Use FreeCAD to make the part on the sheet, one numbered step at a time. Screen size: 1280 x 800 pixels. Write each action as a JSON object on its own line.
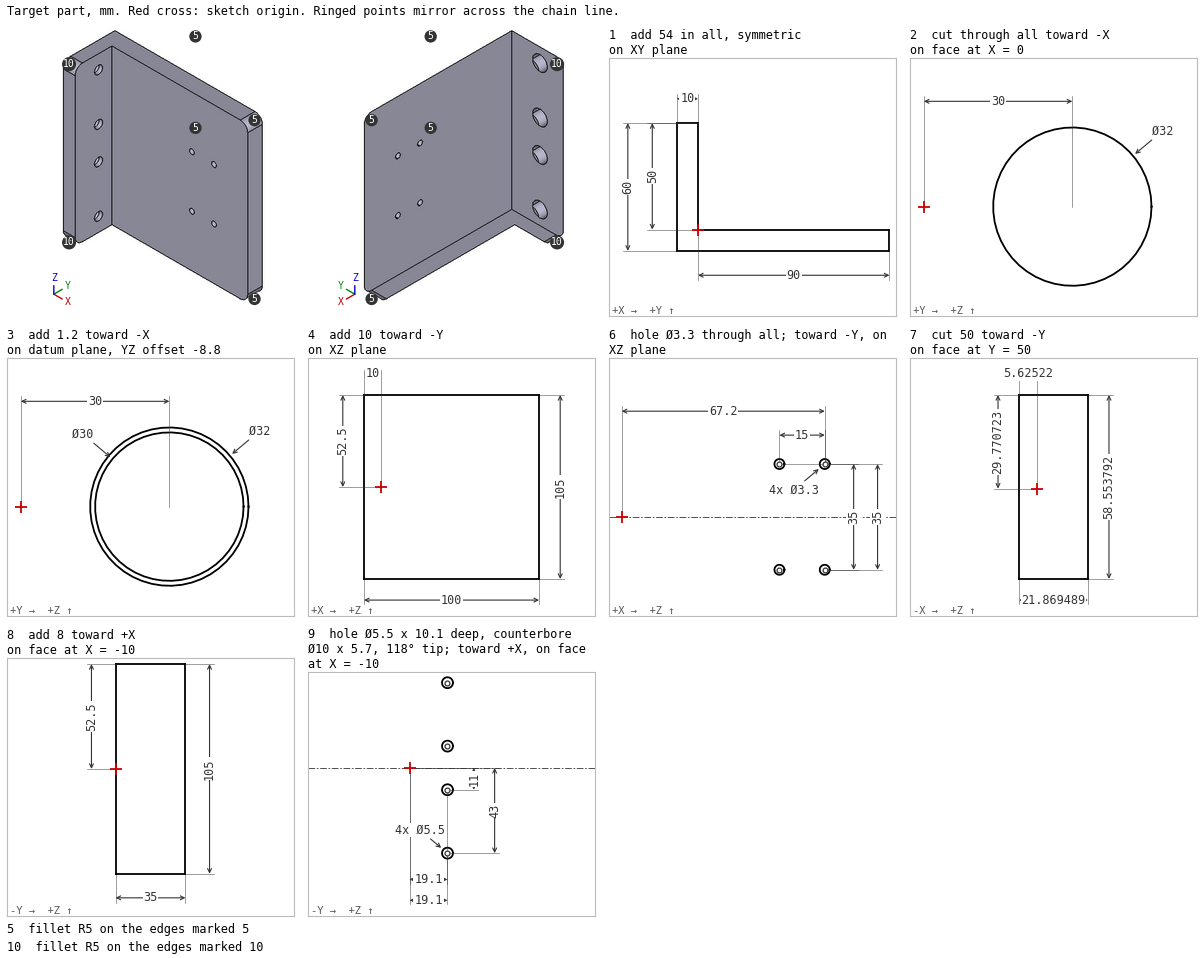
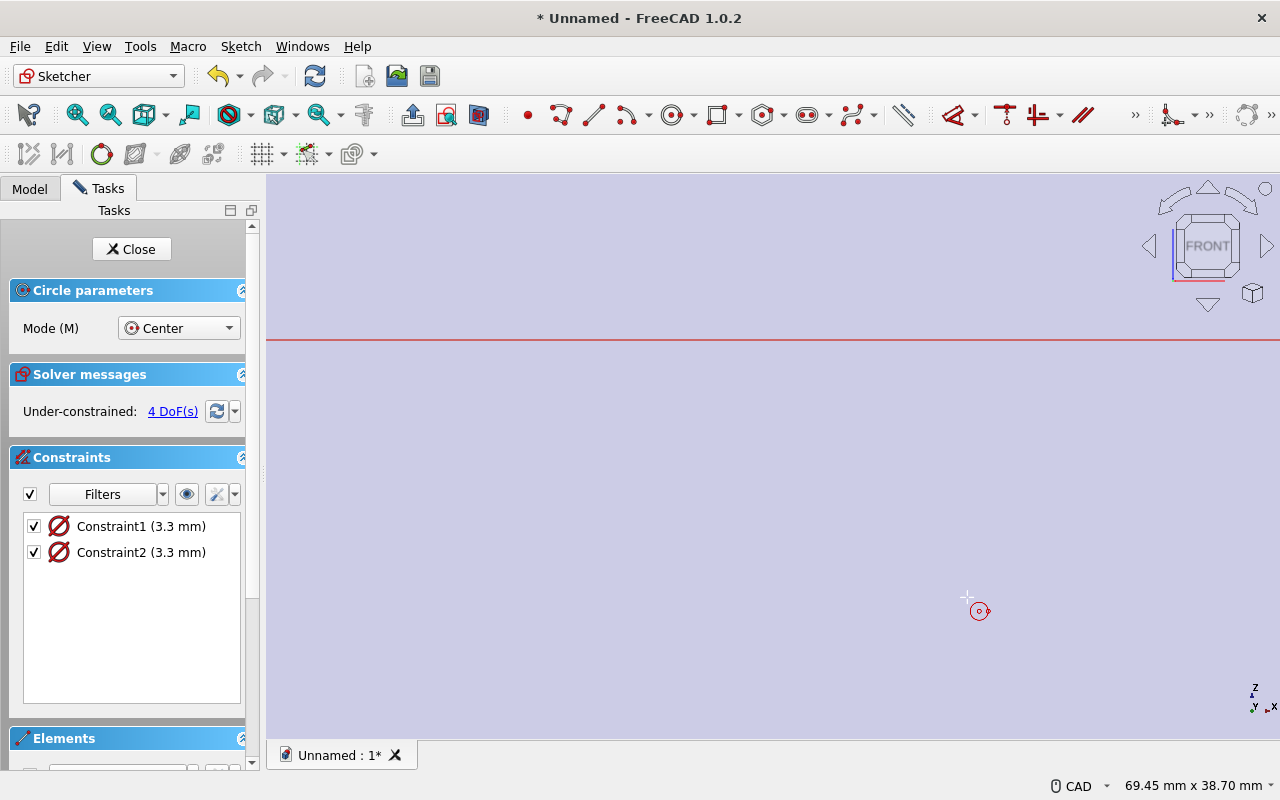
{"action": "left_click", "coordinate": [967, 596]}
{"action": "mouse_move", "coordinate": [984, 579]}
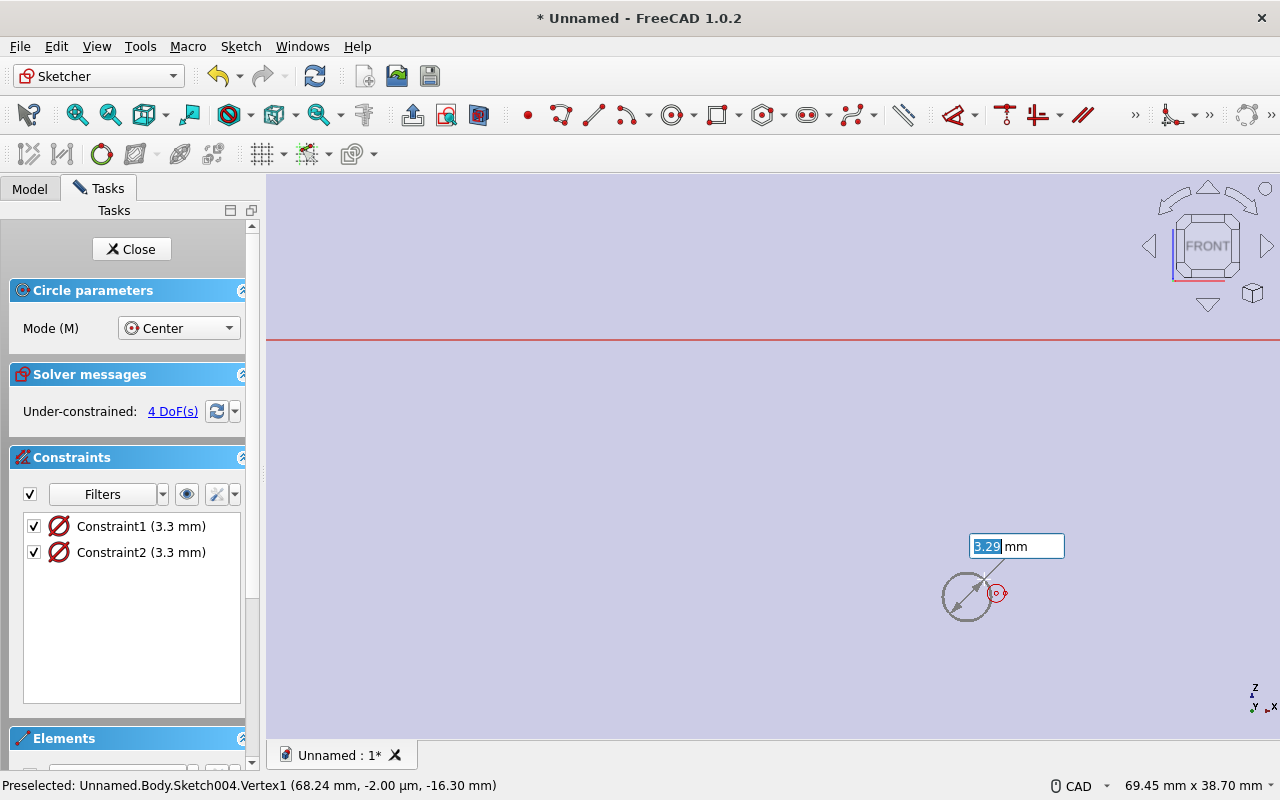
{"action": "type", "text": "3.3"}
{"action": "key", "text": "Return"}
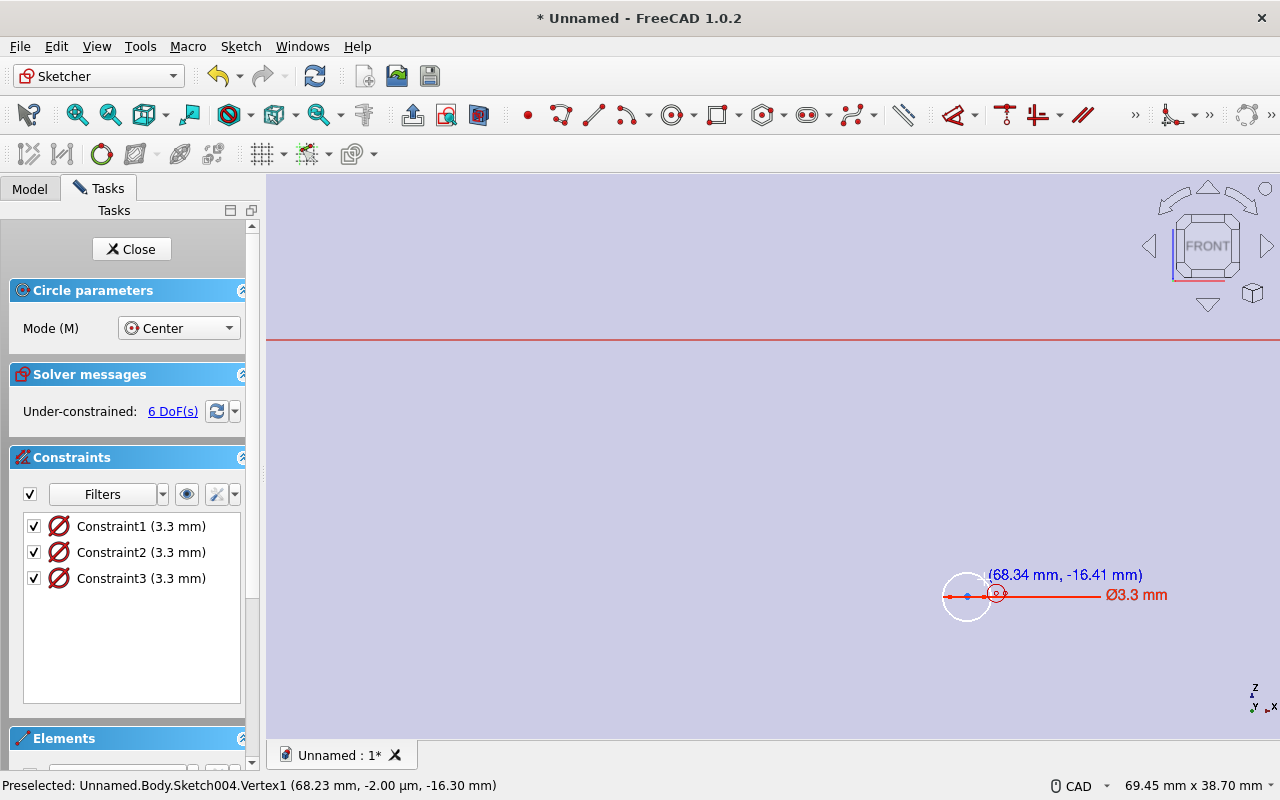
{"action": "left_click", "coordinate": [748, 596]}
{"action": "mouse_move", "coordinate": [765, 579]}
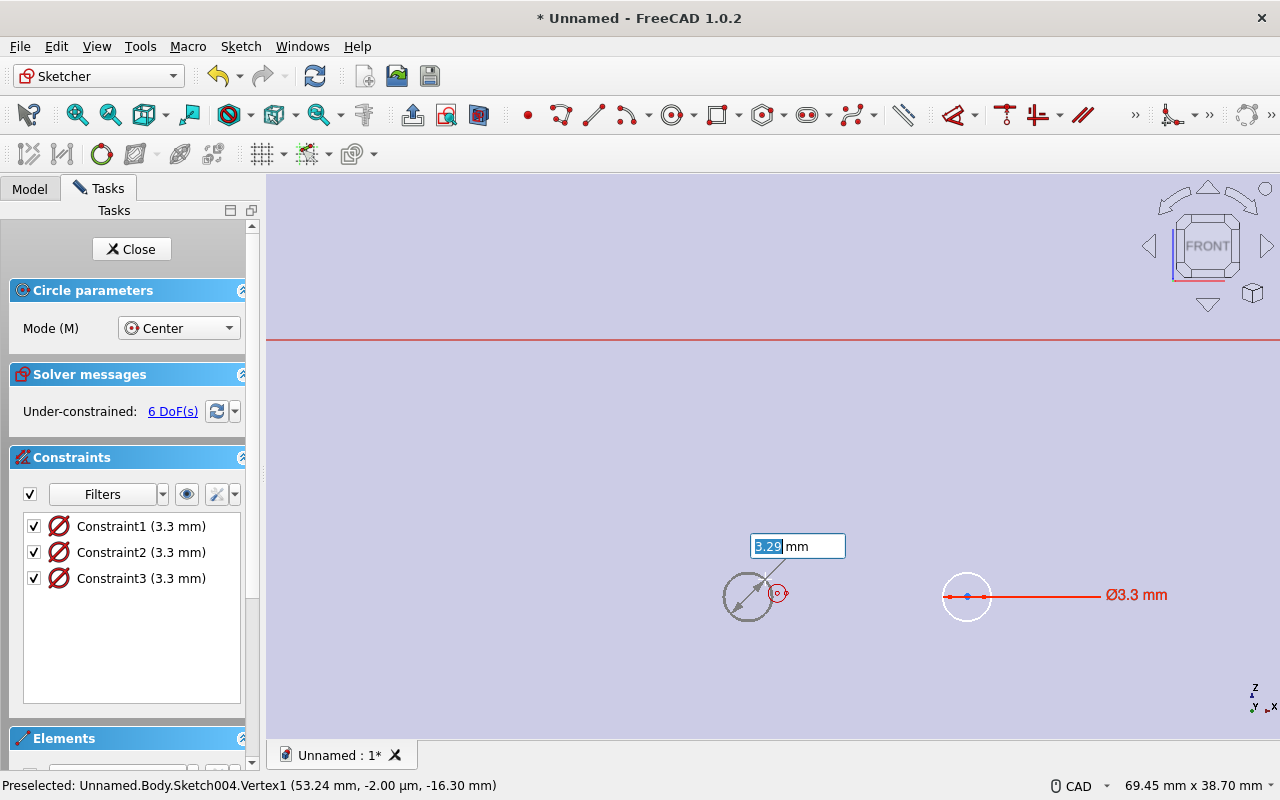
{"action": "type", "text": "3.3"}
{"action": "key", "text": "Return"}
{"action": "key", "text": "Escape"}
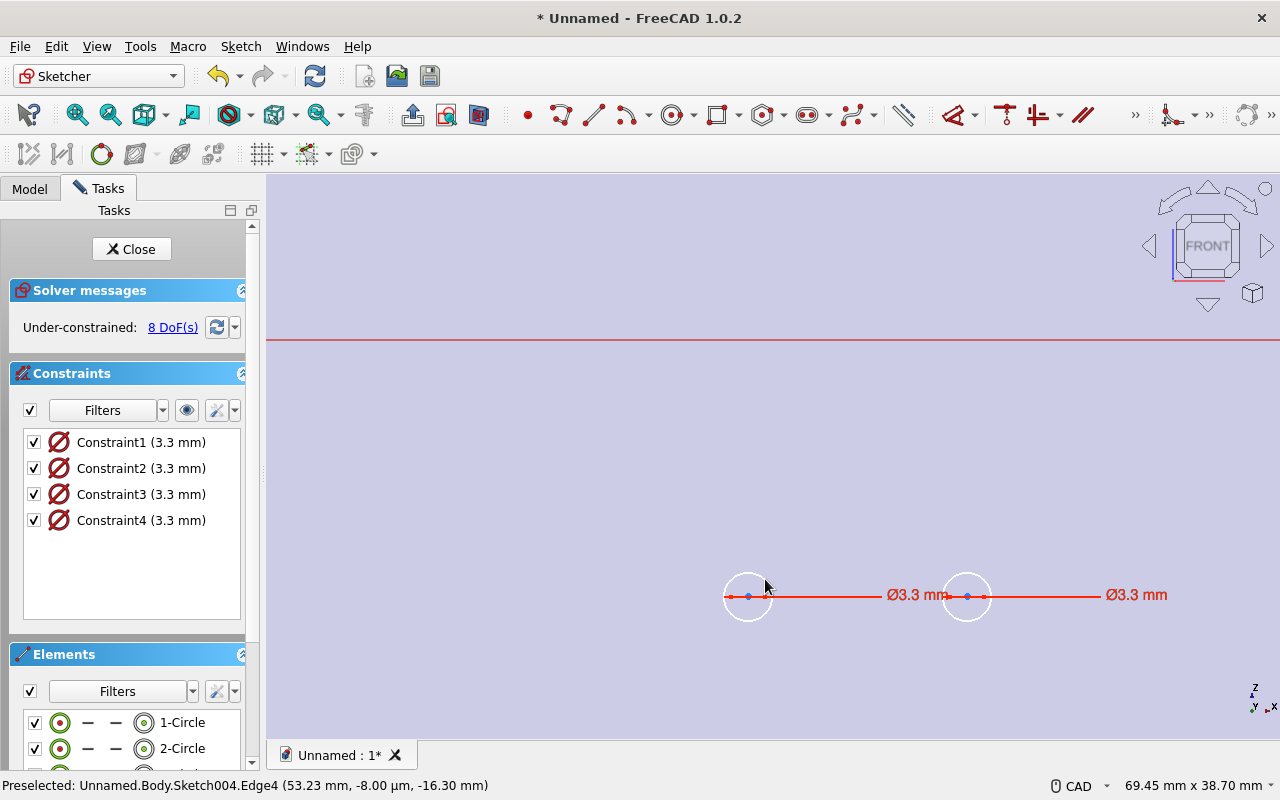
{"action": "scroll", "coordinate": [967, 598], "scroll_direction": "down", "scroll_amount": 3}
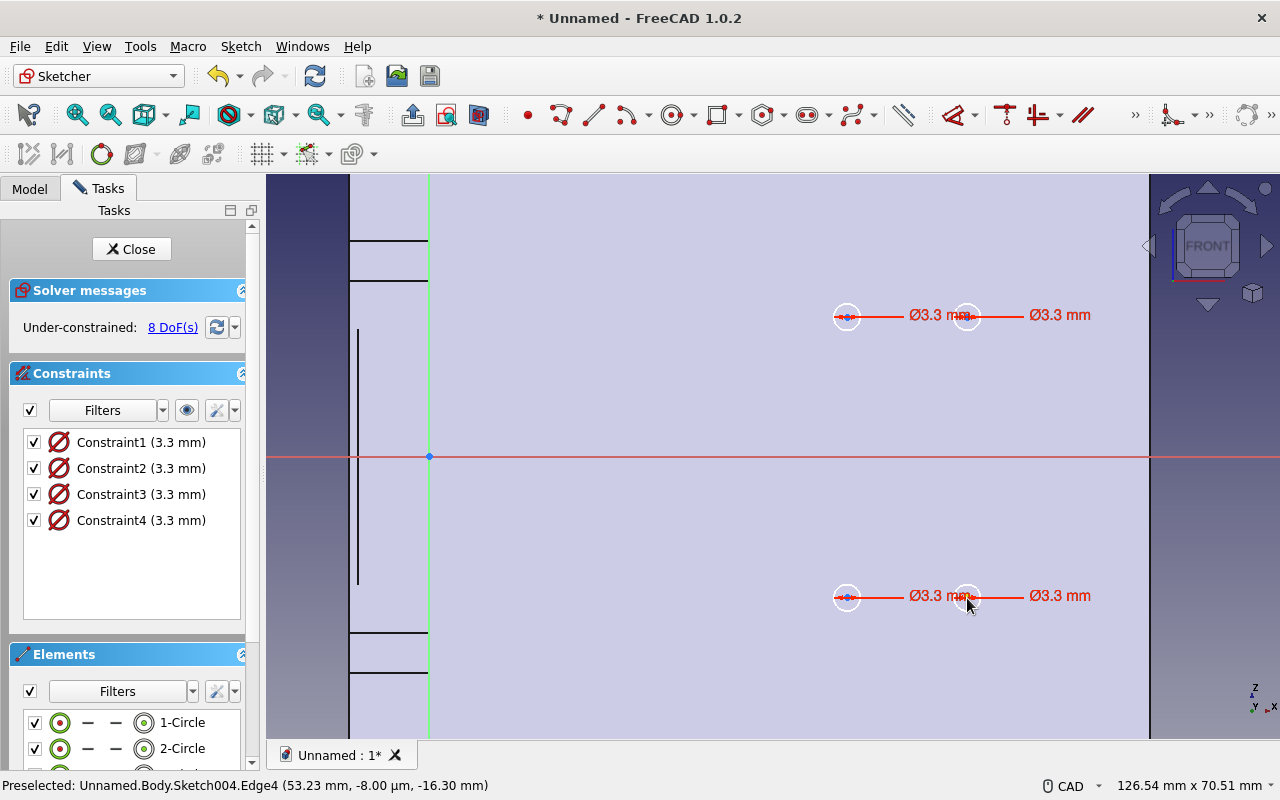
{"action": "left_click", "coordinate": [967, 317]}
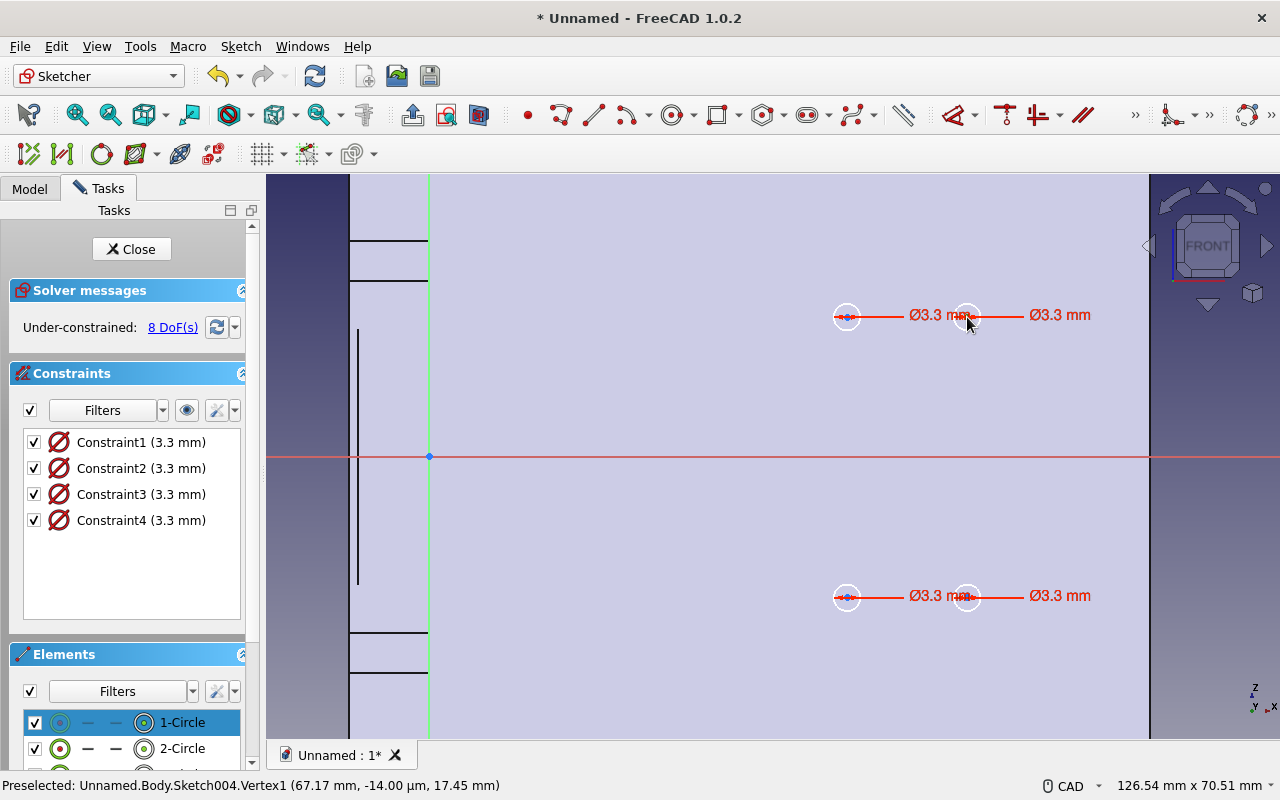
{"action": "left_click", "coordinate": [967, 598]}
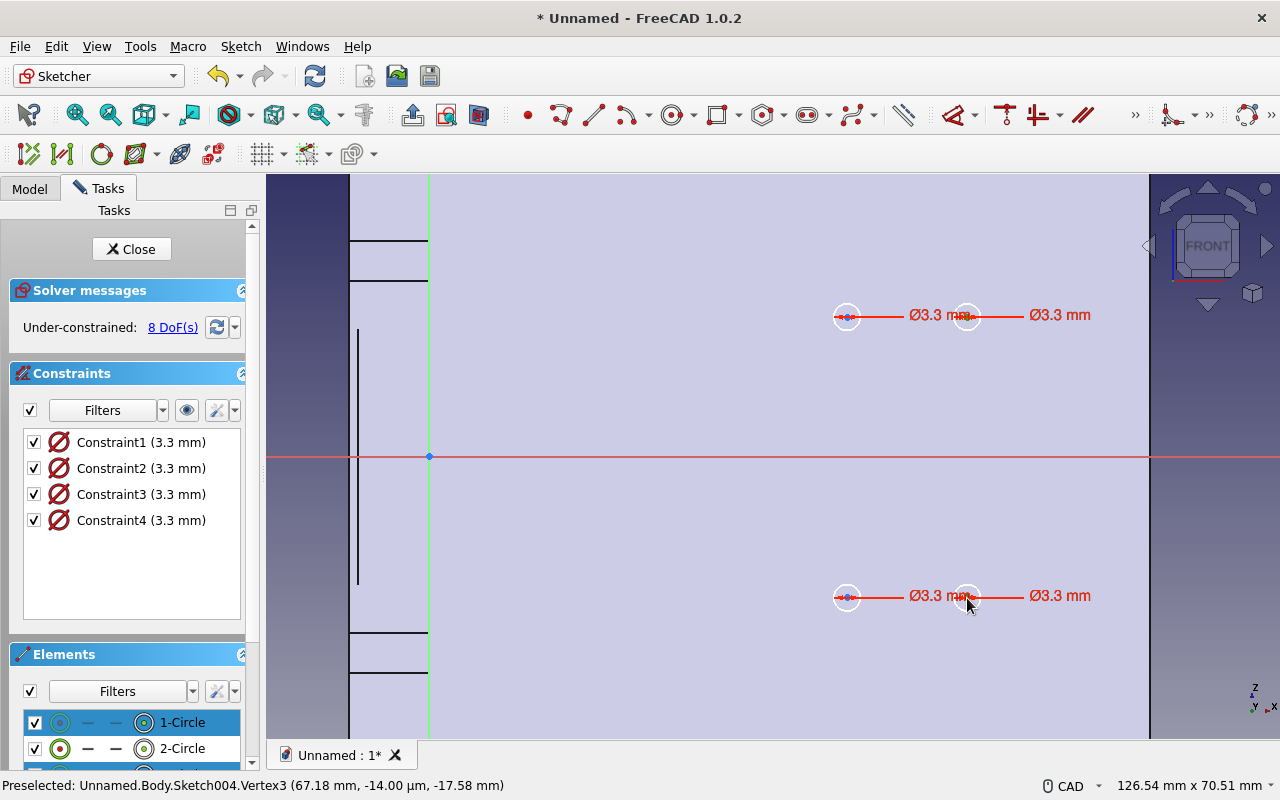
{"action": "left_click", "coordinate": [353, 457]}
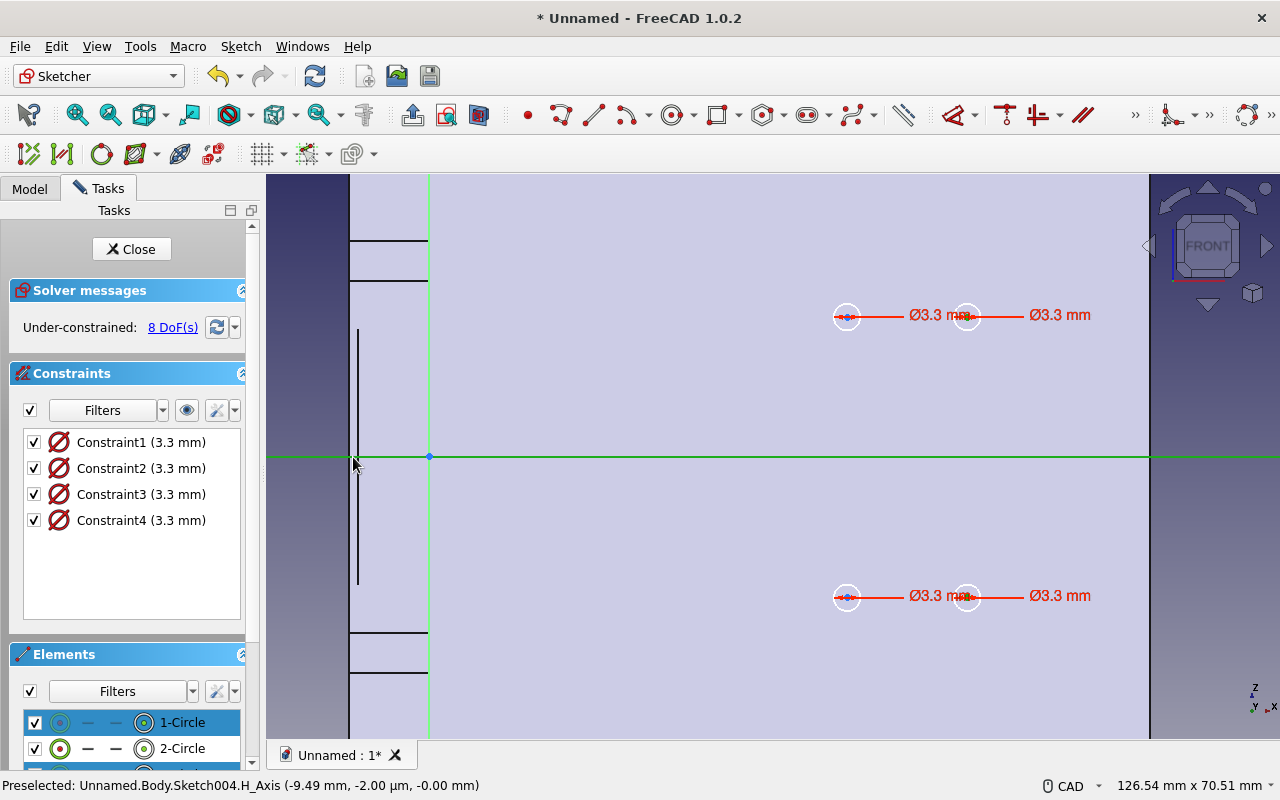
{"action": "key", "text": "s"}